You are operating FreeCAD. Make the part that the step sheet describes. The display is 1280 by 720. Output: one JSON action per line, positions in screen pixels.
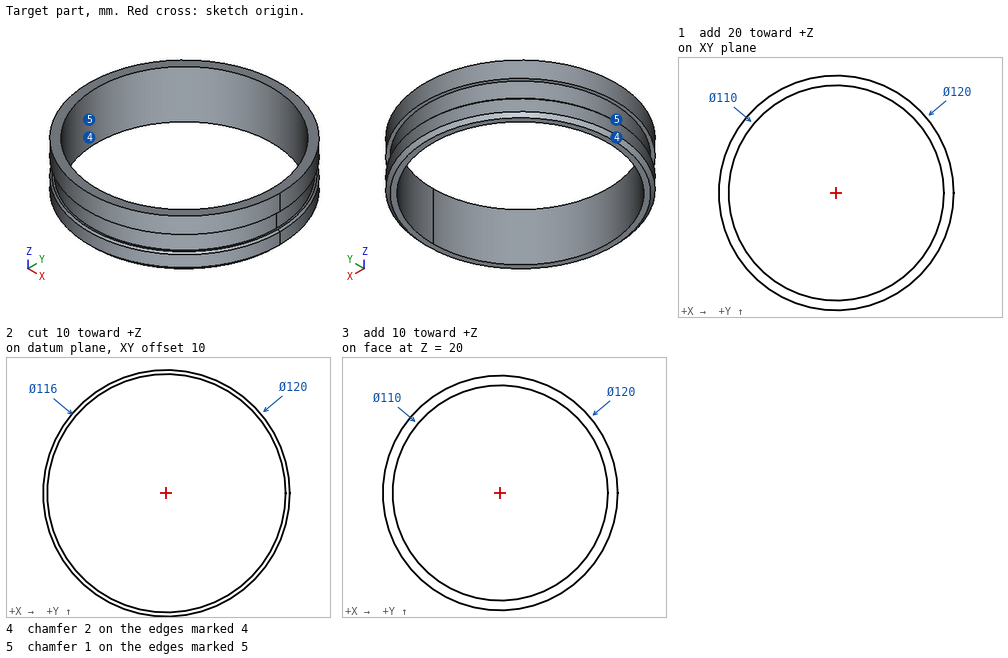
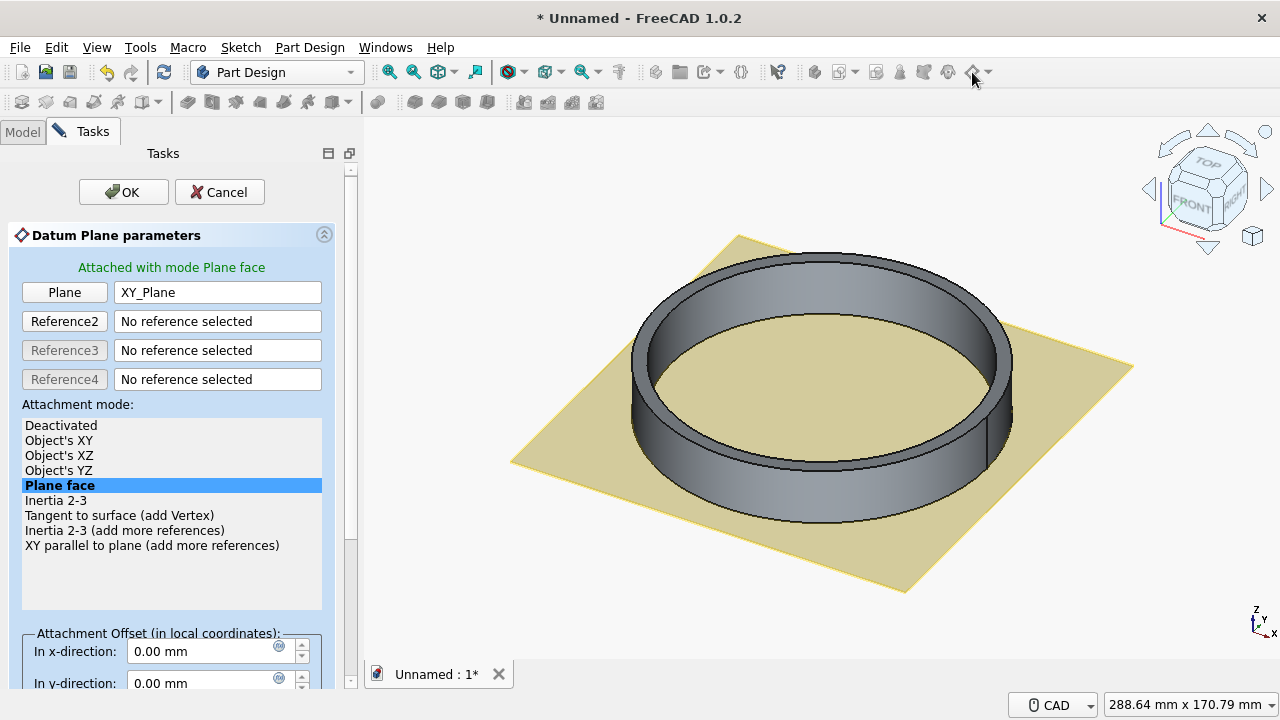
{"action": "scroll", "coordinate": [351, 426], "scroll_direction": "down", "scroll_amount": 2}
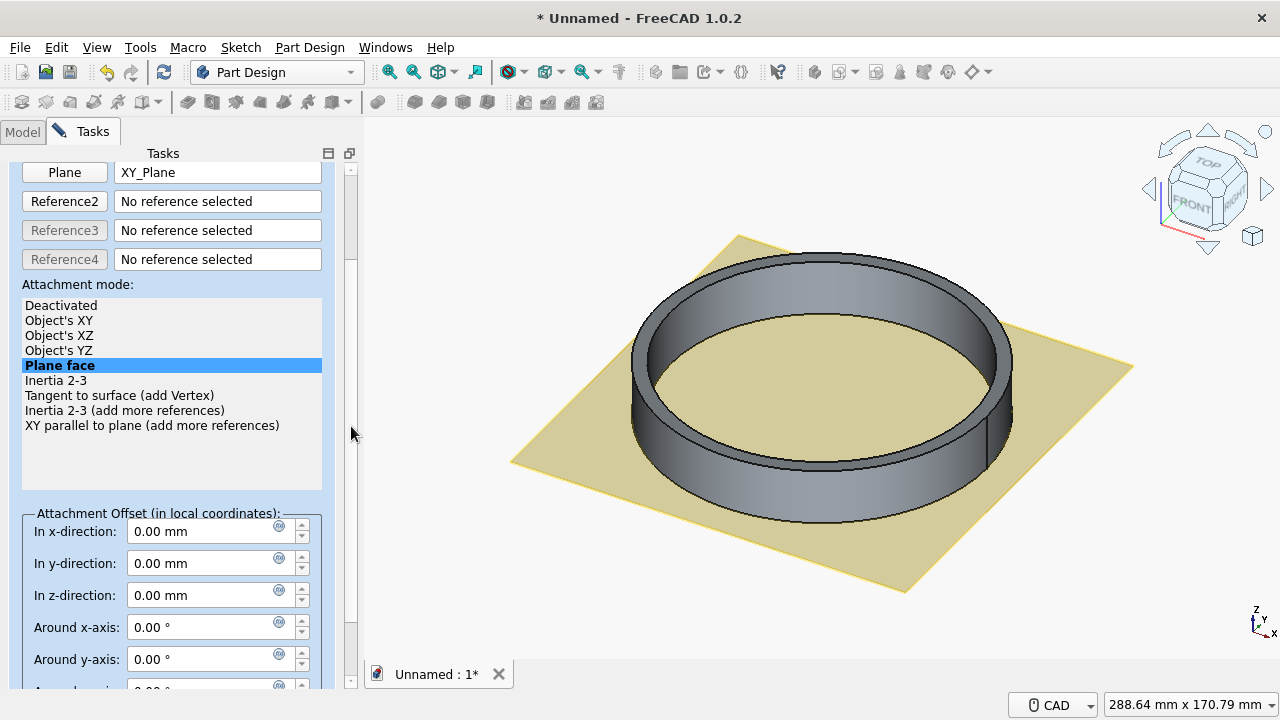
{"action": "triple_click", "coordinate": [210, 595]}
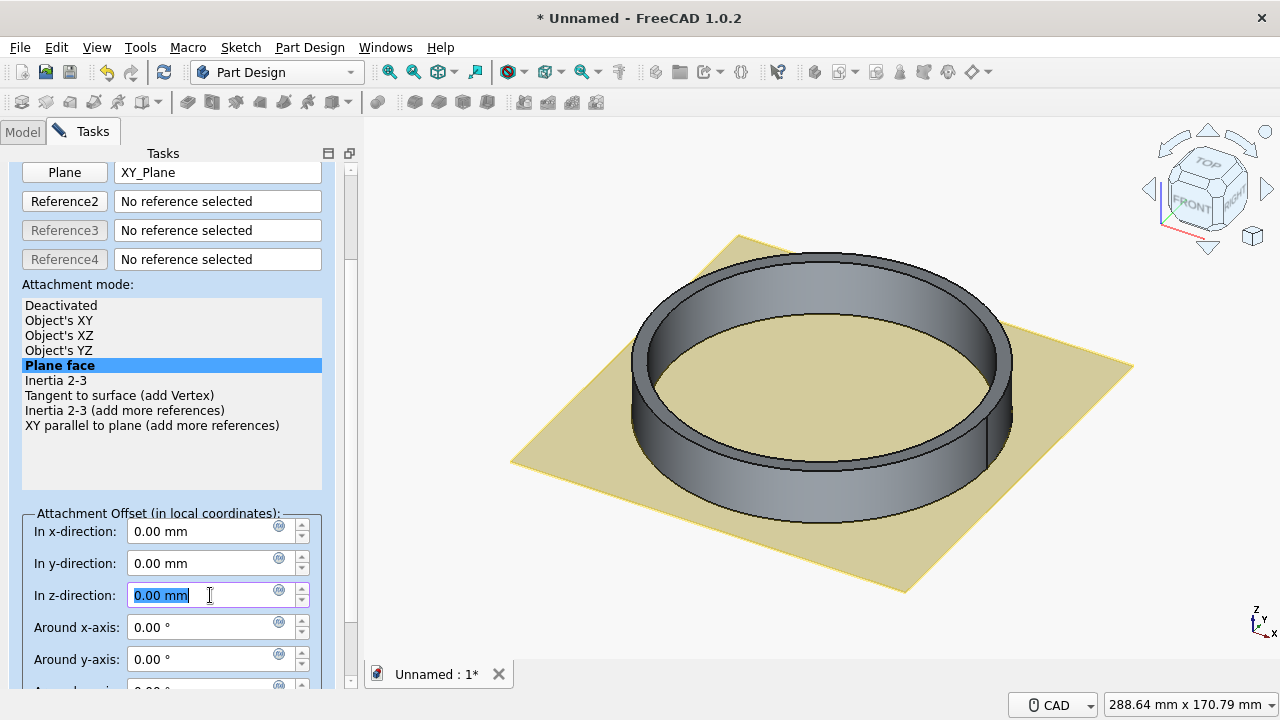
{"action": "type", "text": "10"}
{"action": "key", "text": "Tab"}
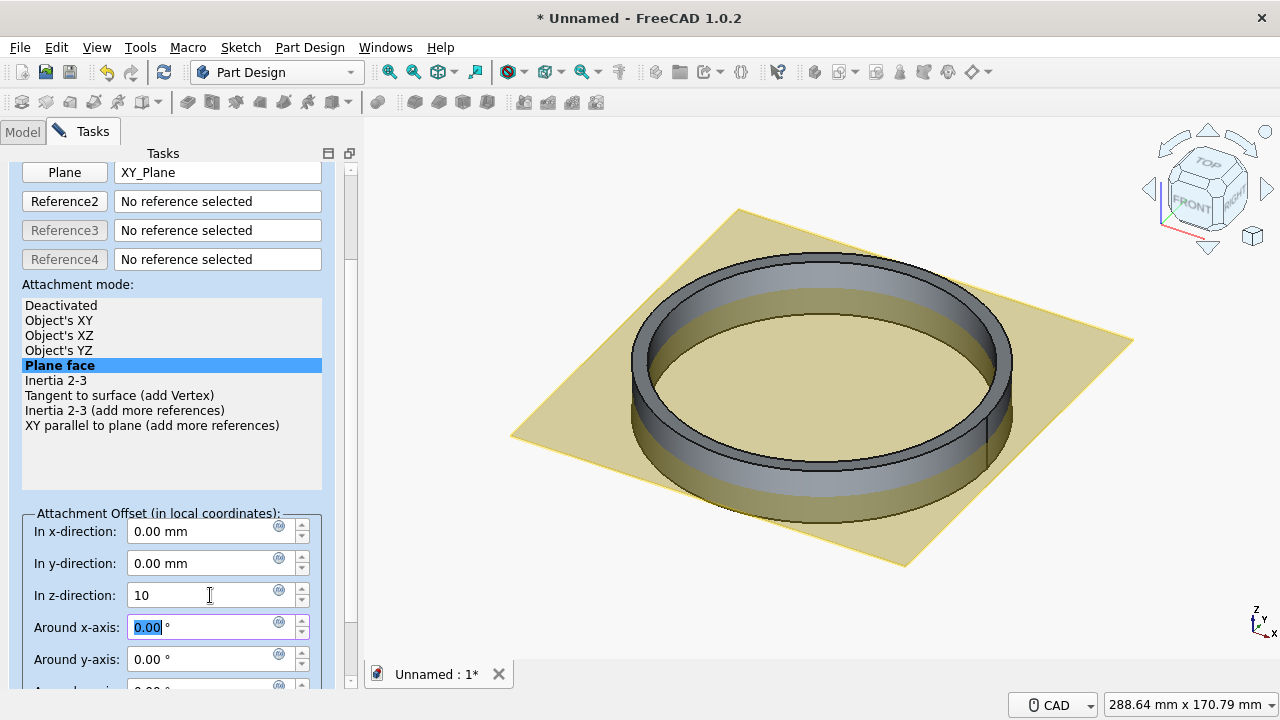
{"action": "scroll", "coordinate": [351, 426], "scroll_direction": "up", "scroll_amount": 3}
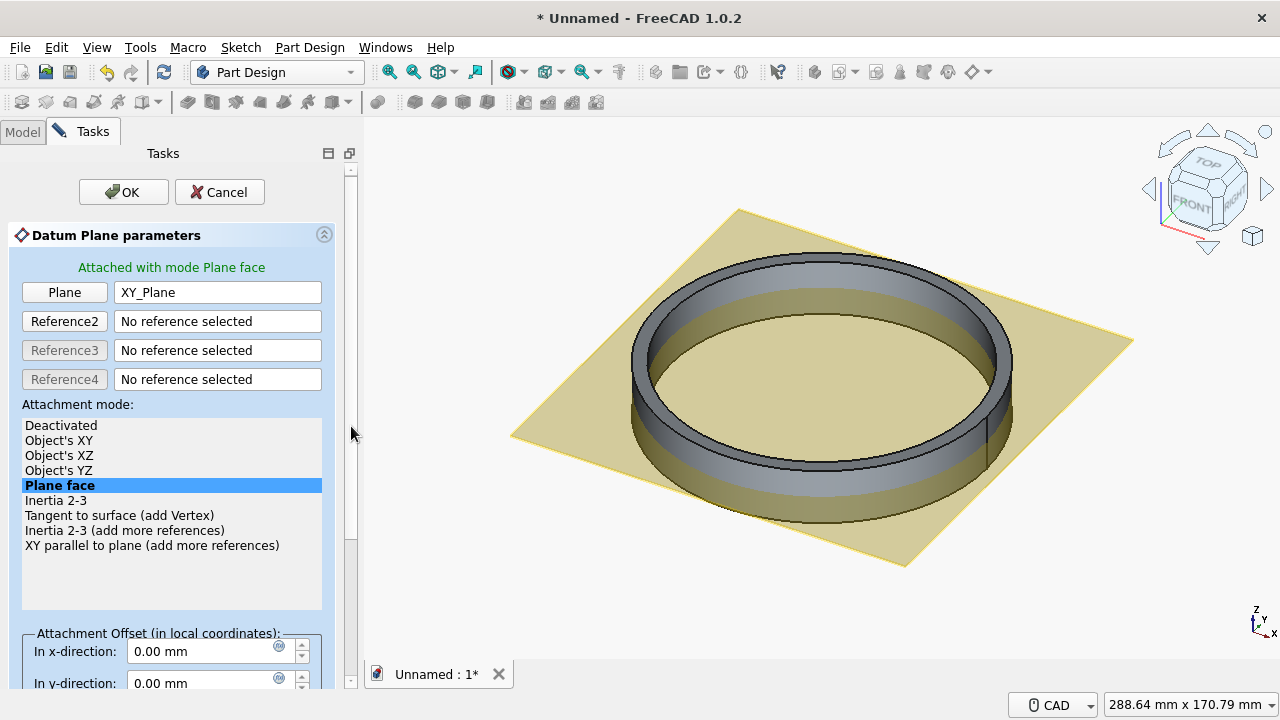
{"action": "left_click", "coordinate": [124, 192]}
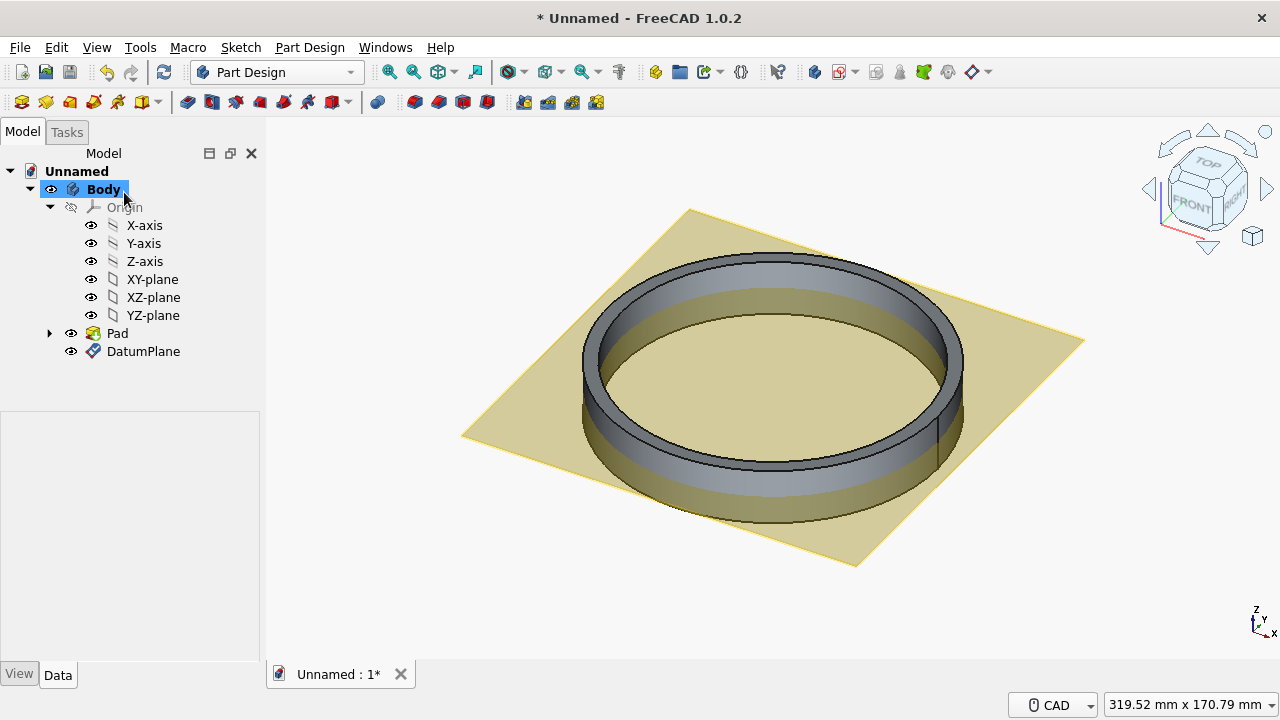
{"action": "left_click", "coordinate": [116, 351]}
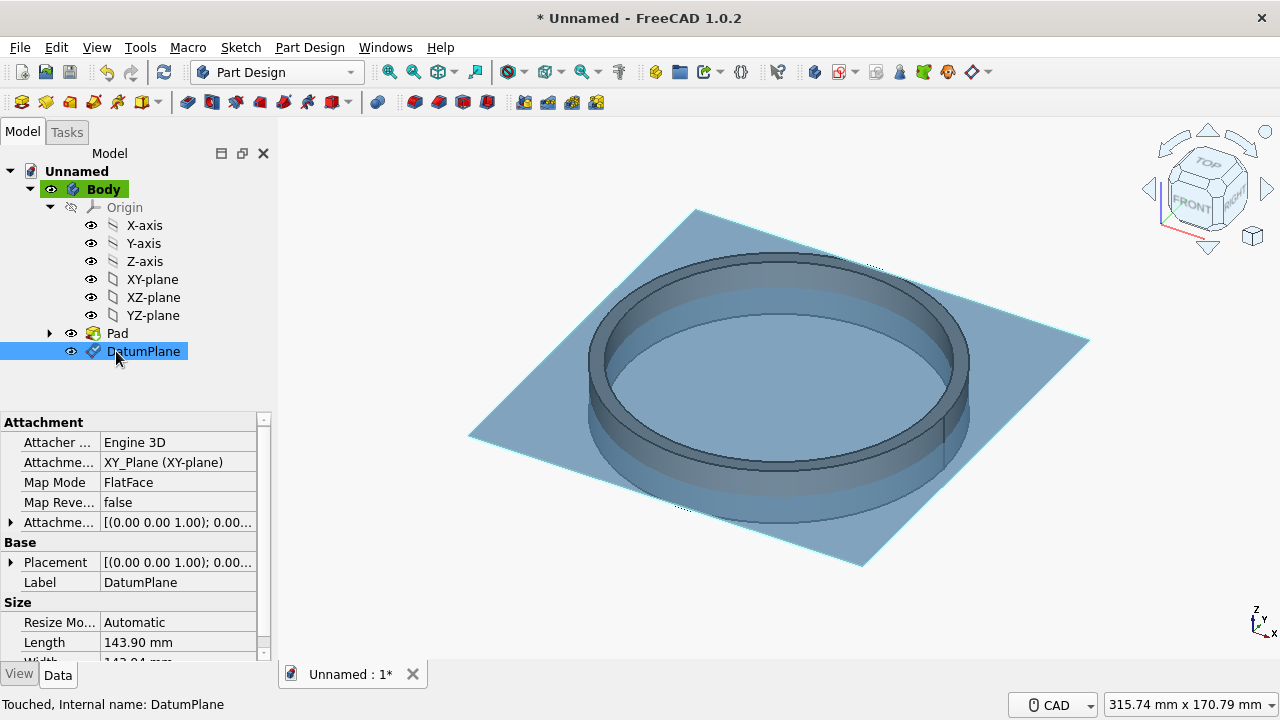
{"action": "left_click", "coordinate": [840, 72]}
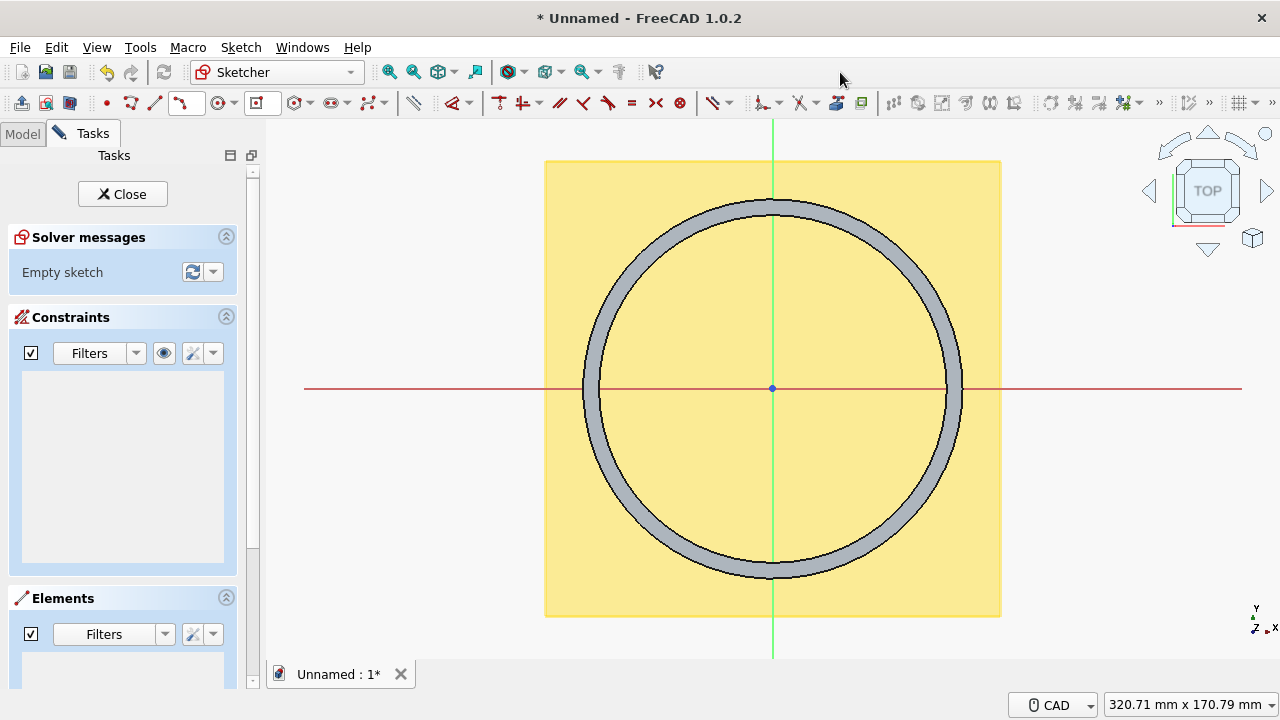
{"action": "key", "text": "q s"}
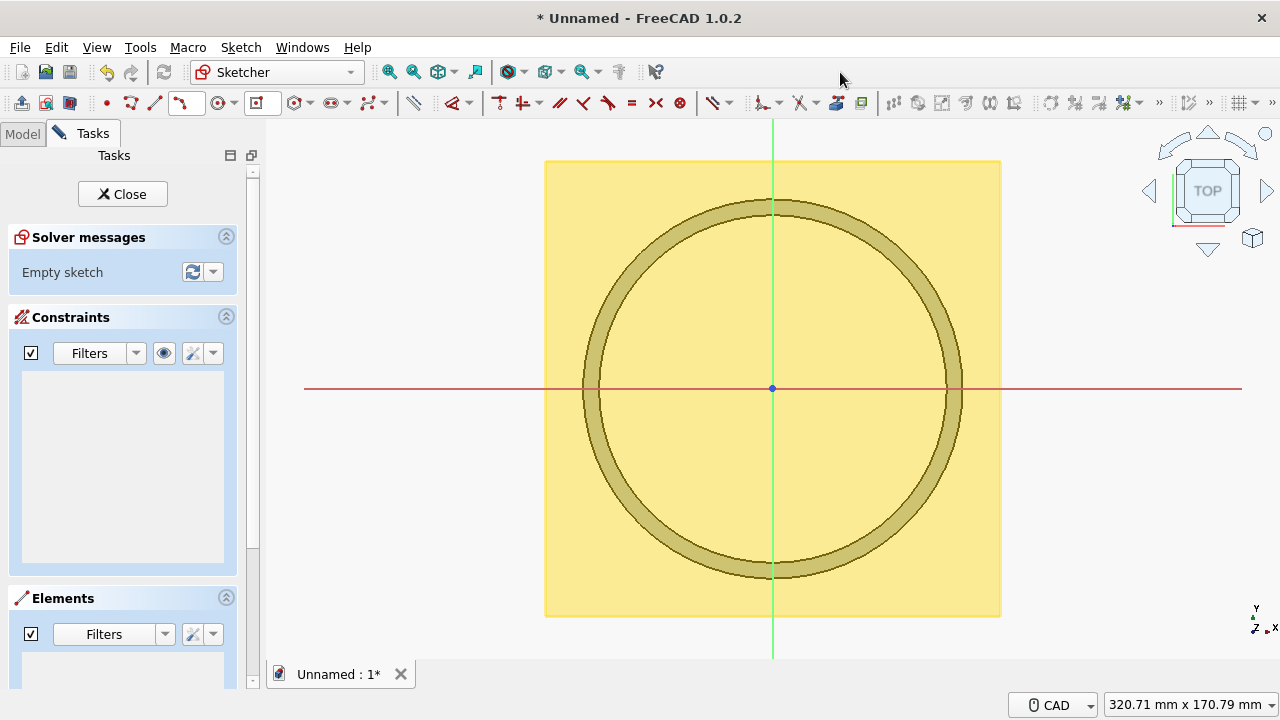
{"action": "left_click", "coordinate": [218, 104]}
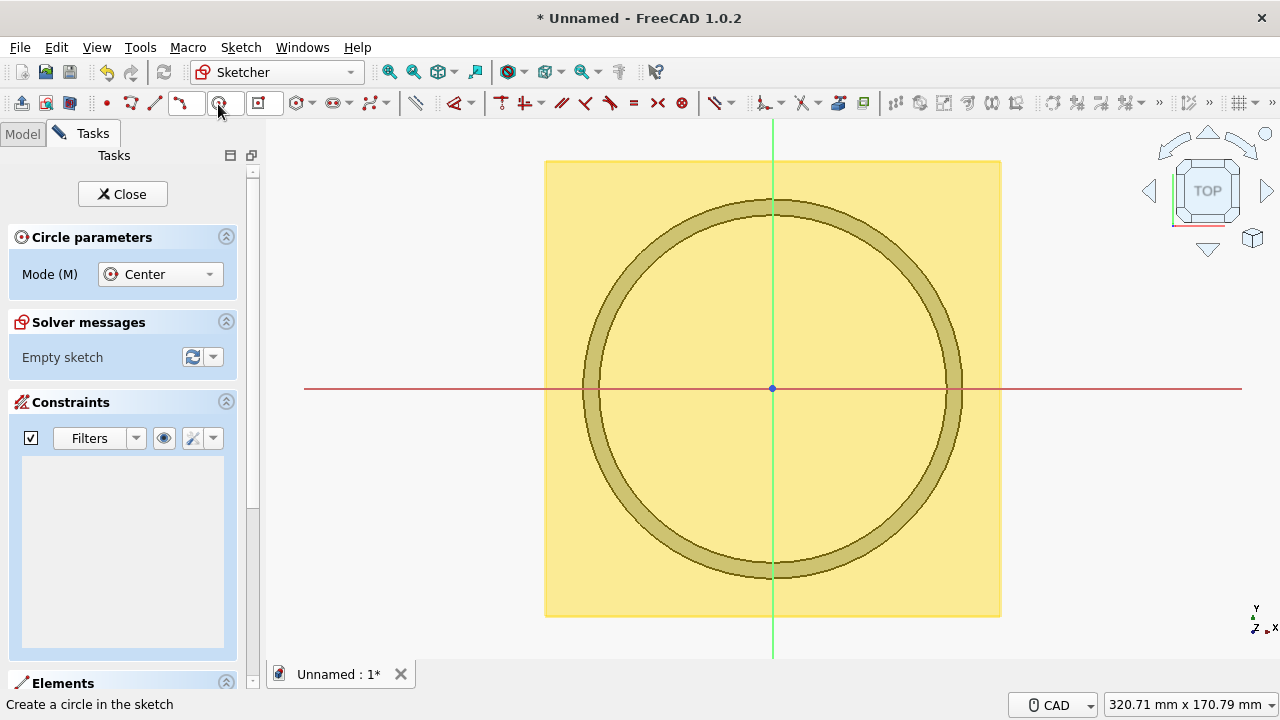
{"action": "left_click", "coordinate": [773, 389]}
{"action": "left_click", "coordinate": [907, 255]}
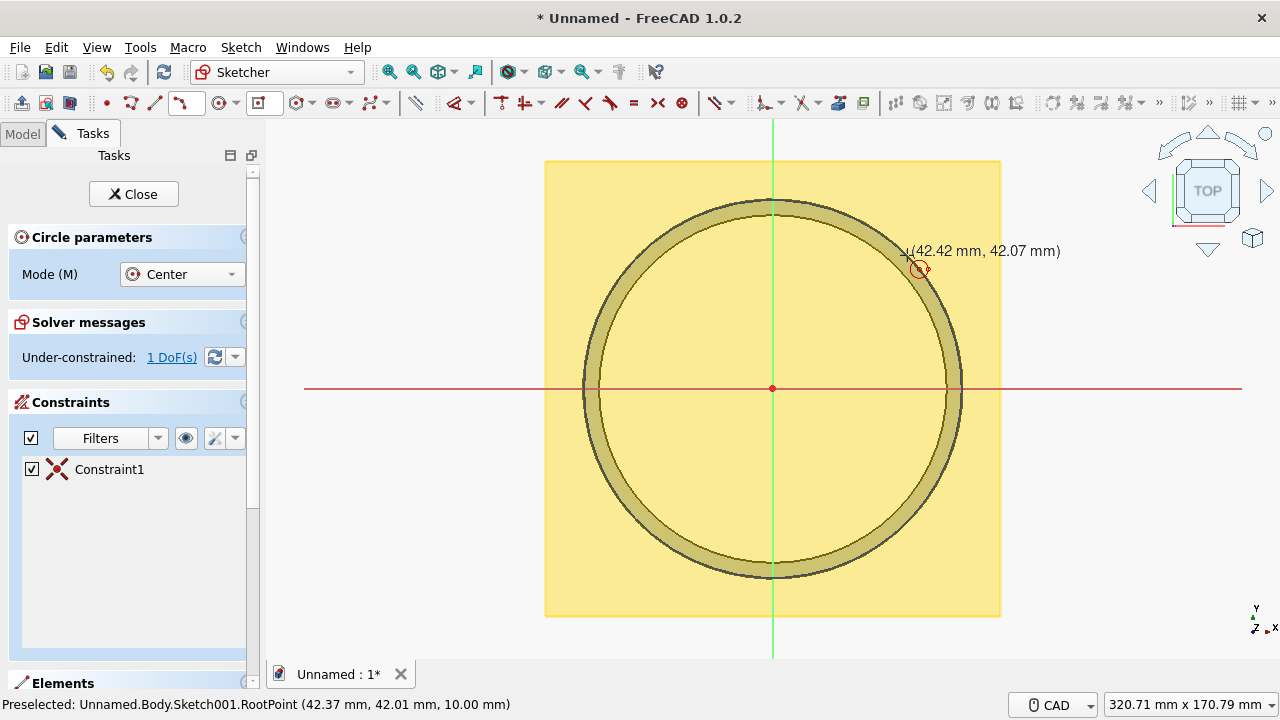
{"action": "left_click", "coordinate": [773, 389]}